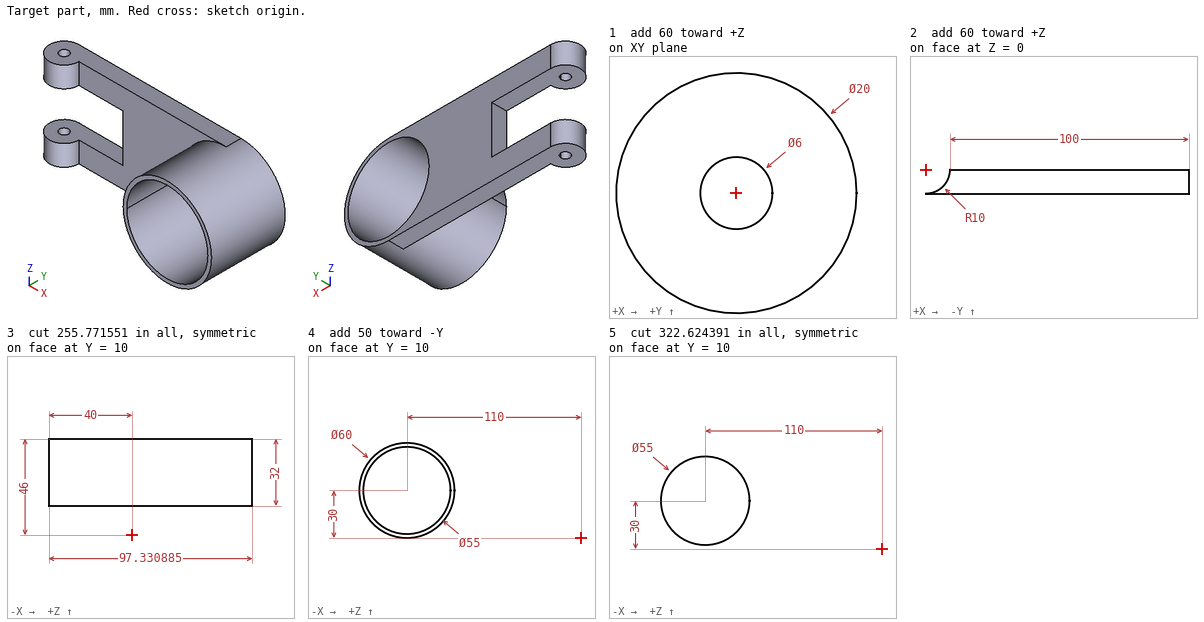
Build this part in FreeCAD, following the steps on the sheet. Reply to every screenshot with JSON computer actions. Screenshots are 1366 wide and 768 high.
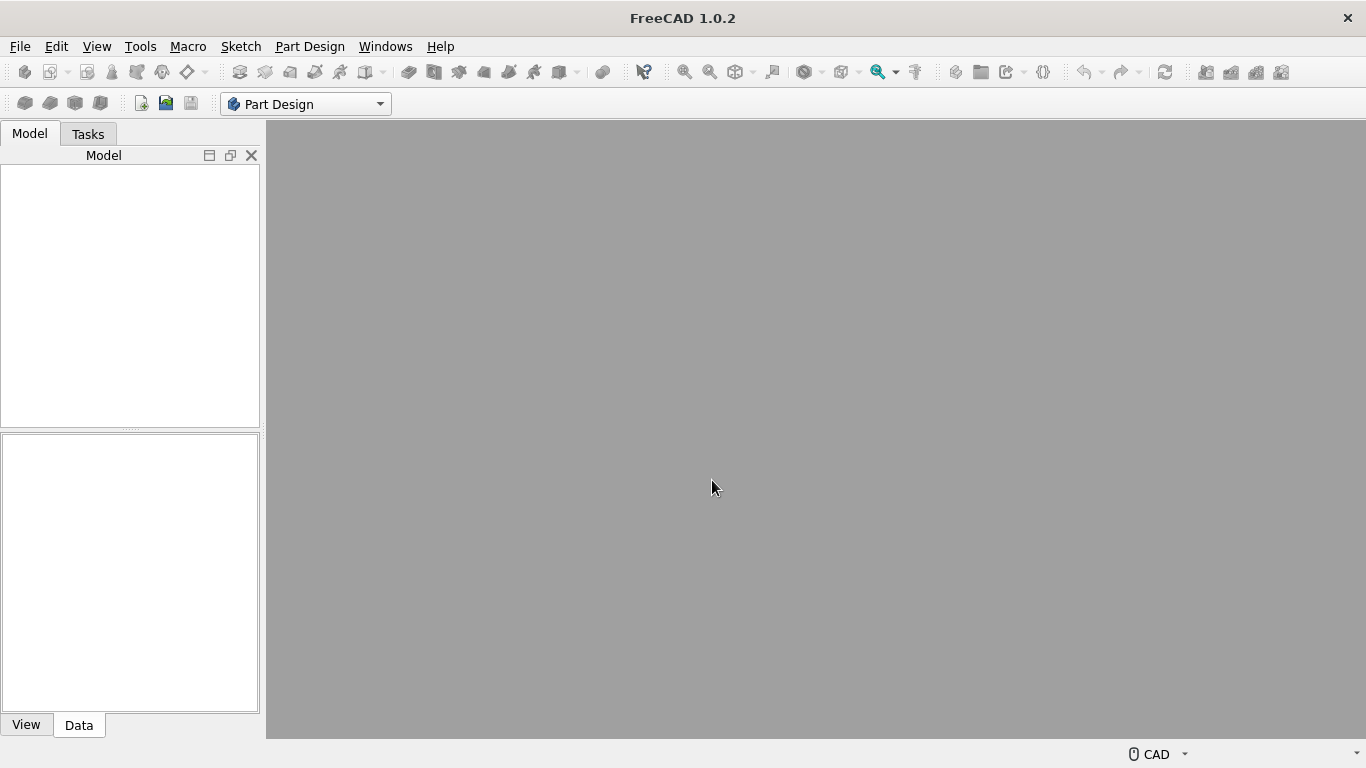
{"action": "left_click", "coordinate": [141, 104]}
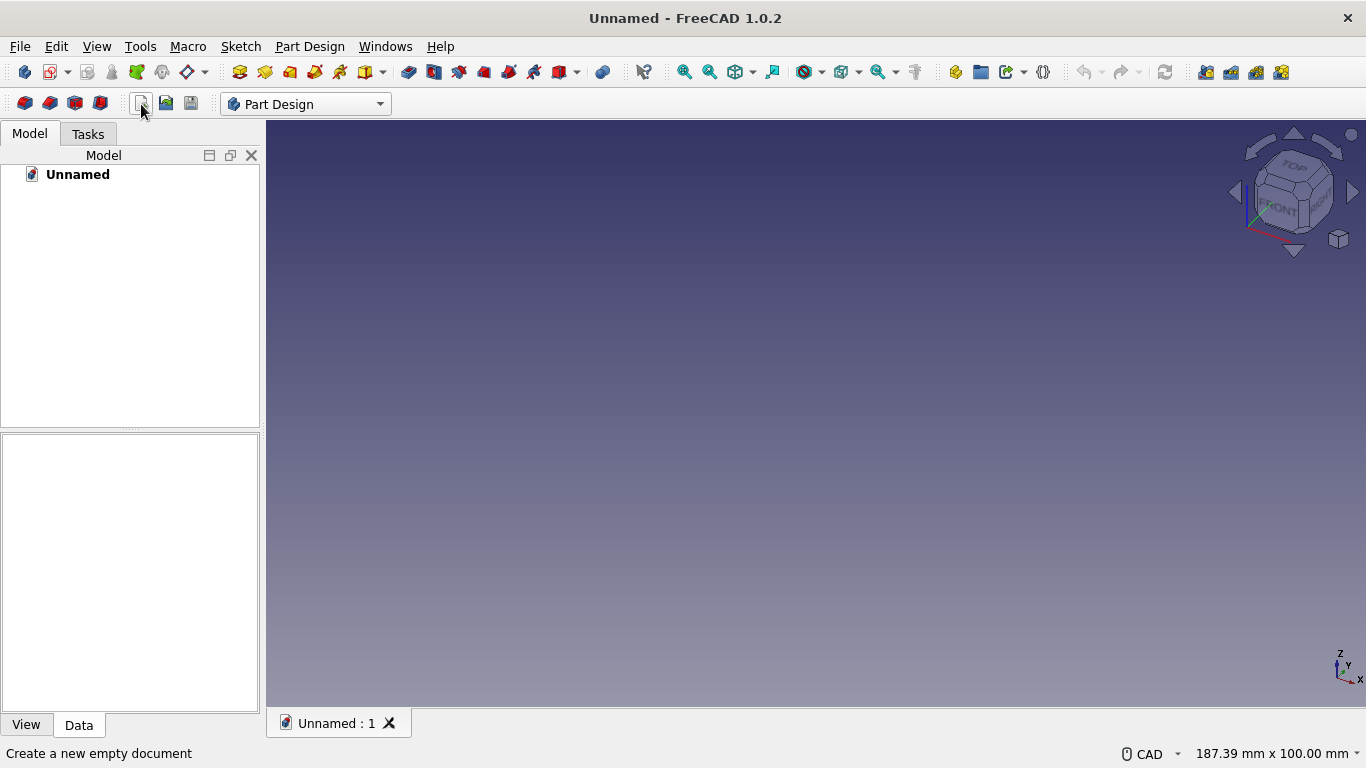
{"action": "left_click", "coordinate": [50, 72]}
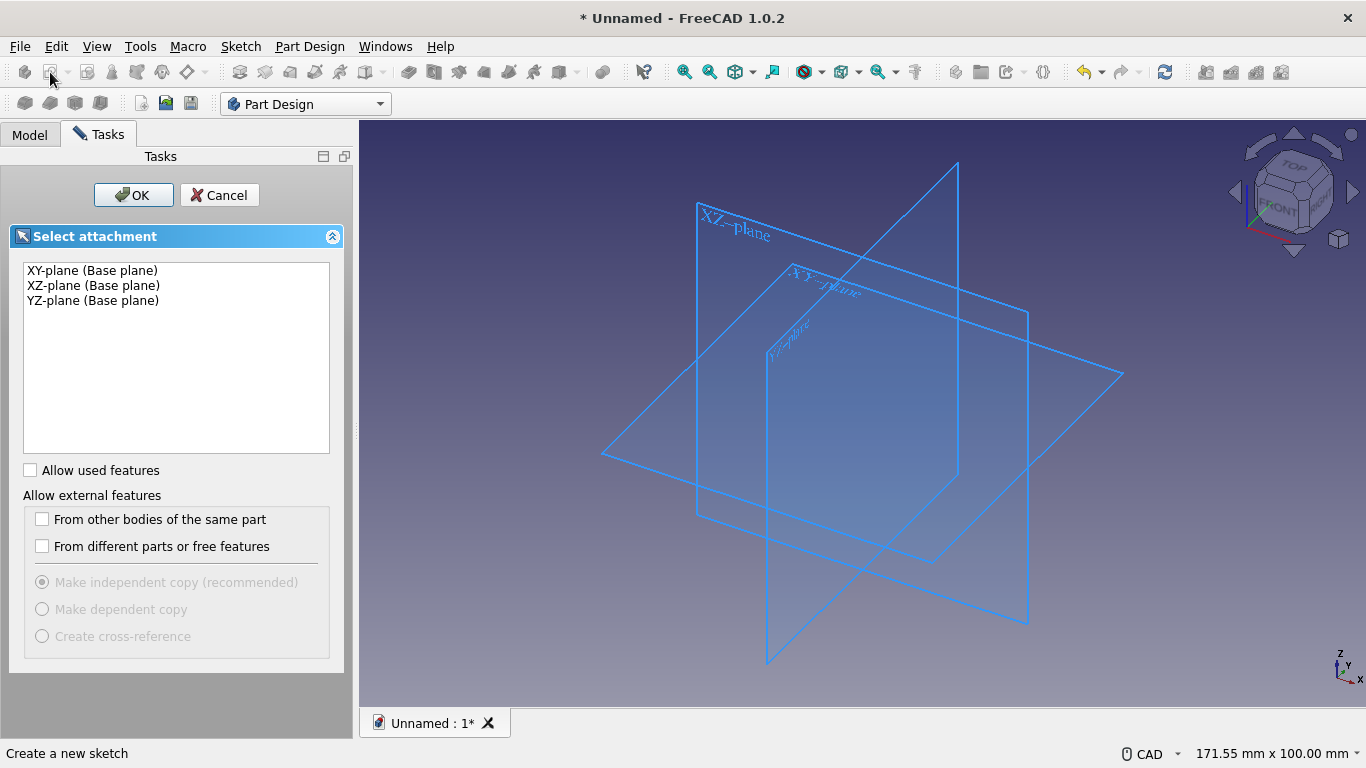
{"action": "left_click", "coordinate": [84, 270]}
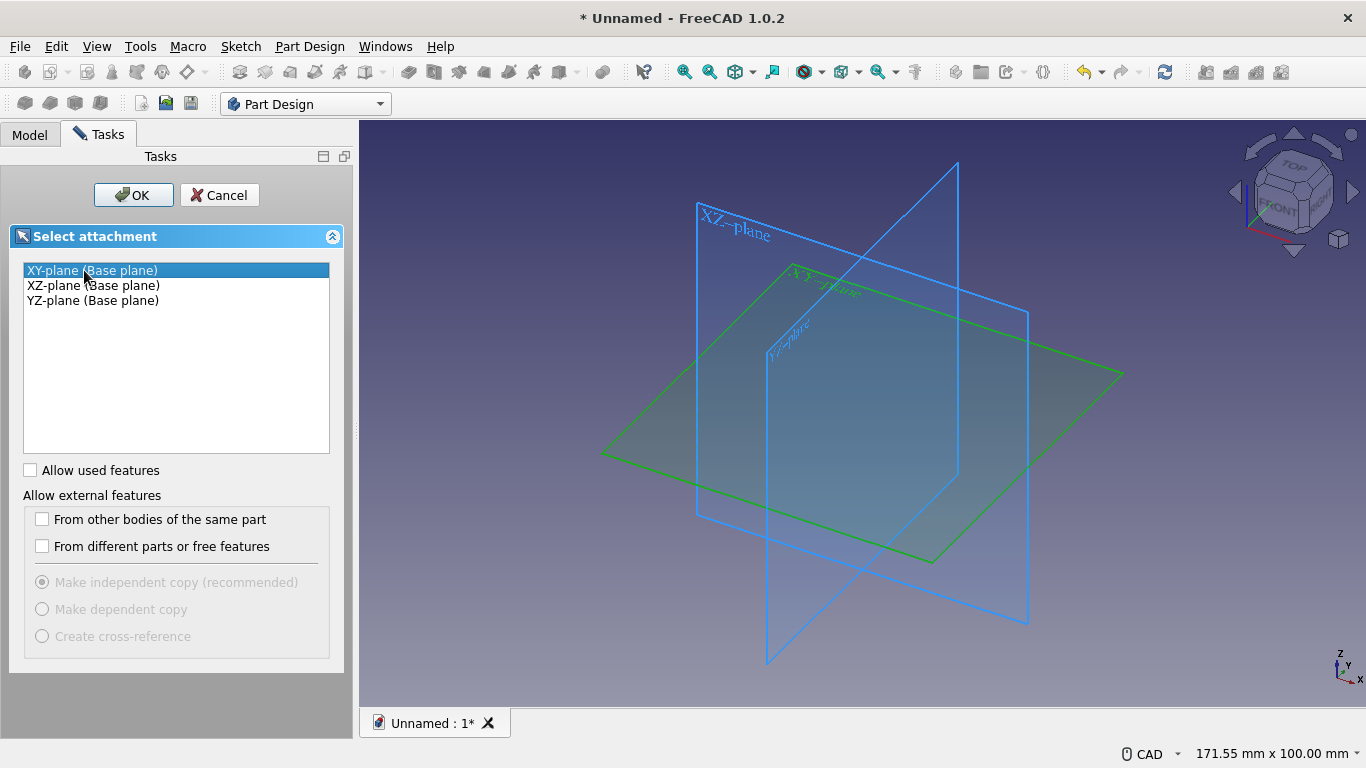
{"action": "left_click", "coordinate": [134, 195]}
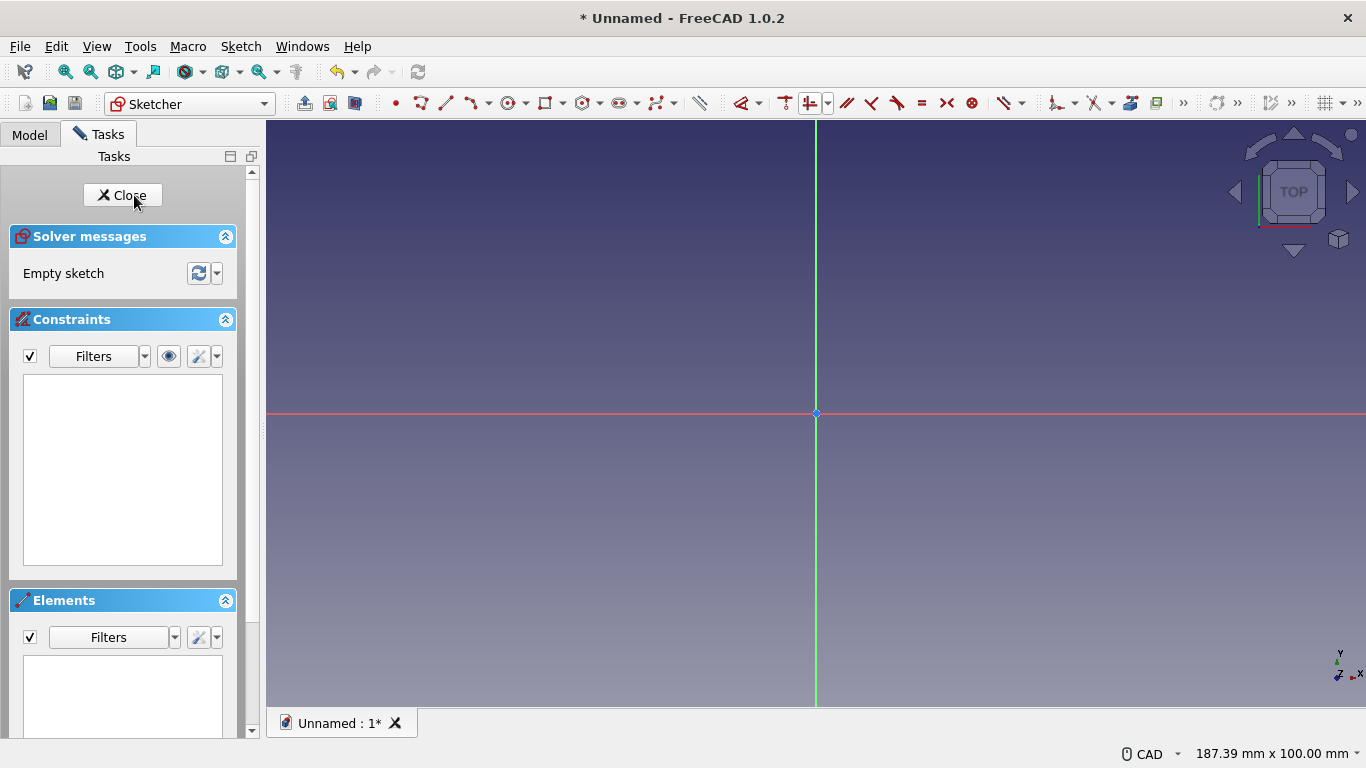
{"action": "scroll", "coordinate": [846, 414], "scroll_direction": "up", "scroll_amount": 6}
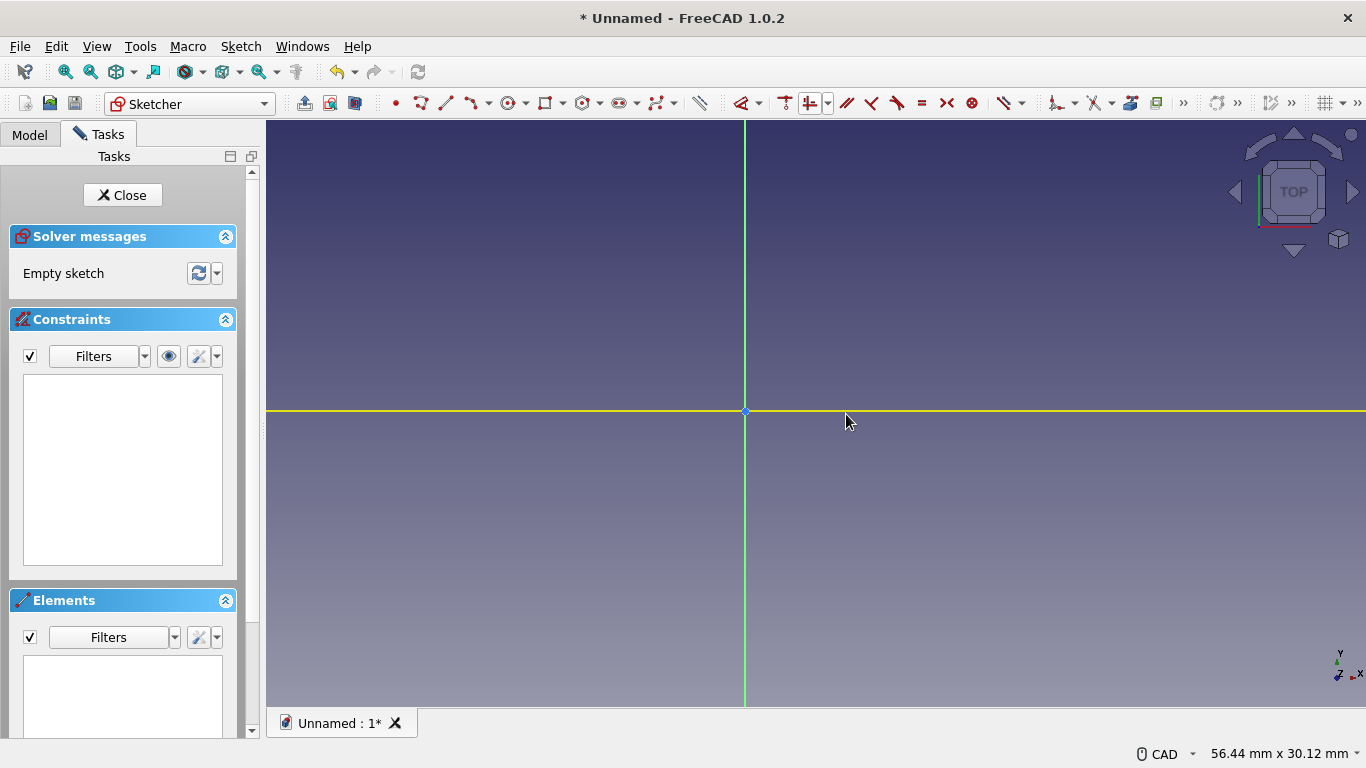
{"action": "left_click", "coordinate": [508, 104]}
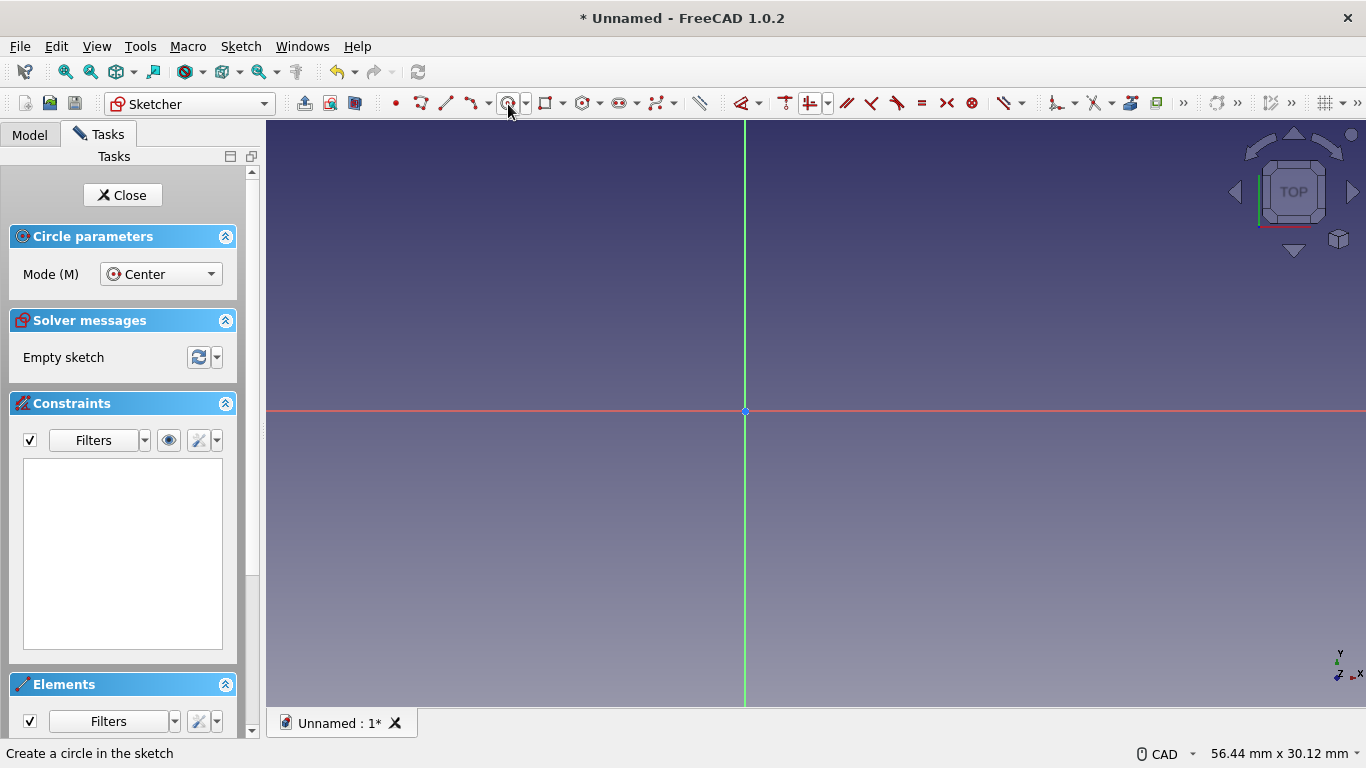
{"action": "left_click", "coordinate": [745, 411]}
{"action": "mouse_move", "coordinate": [883, 273]}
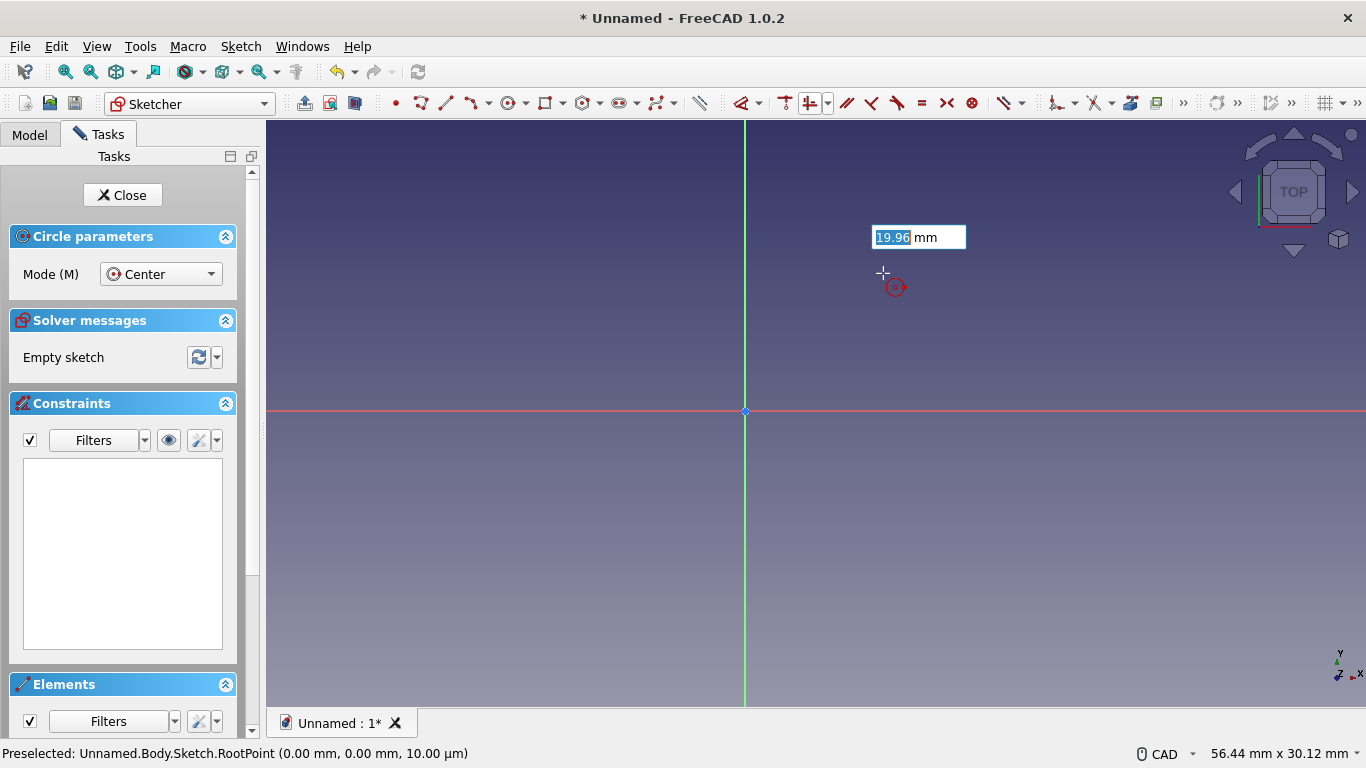
{"action": "type", "text": "20"}
{"action": "key", "text": "Return"}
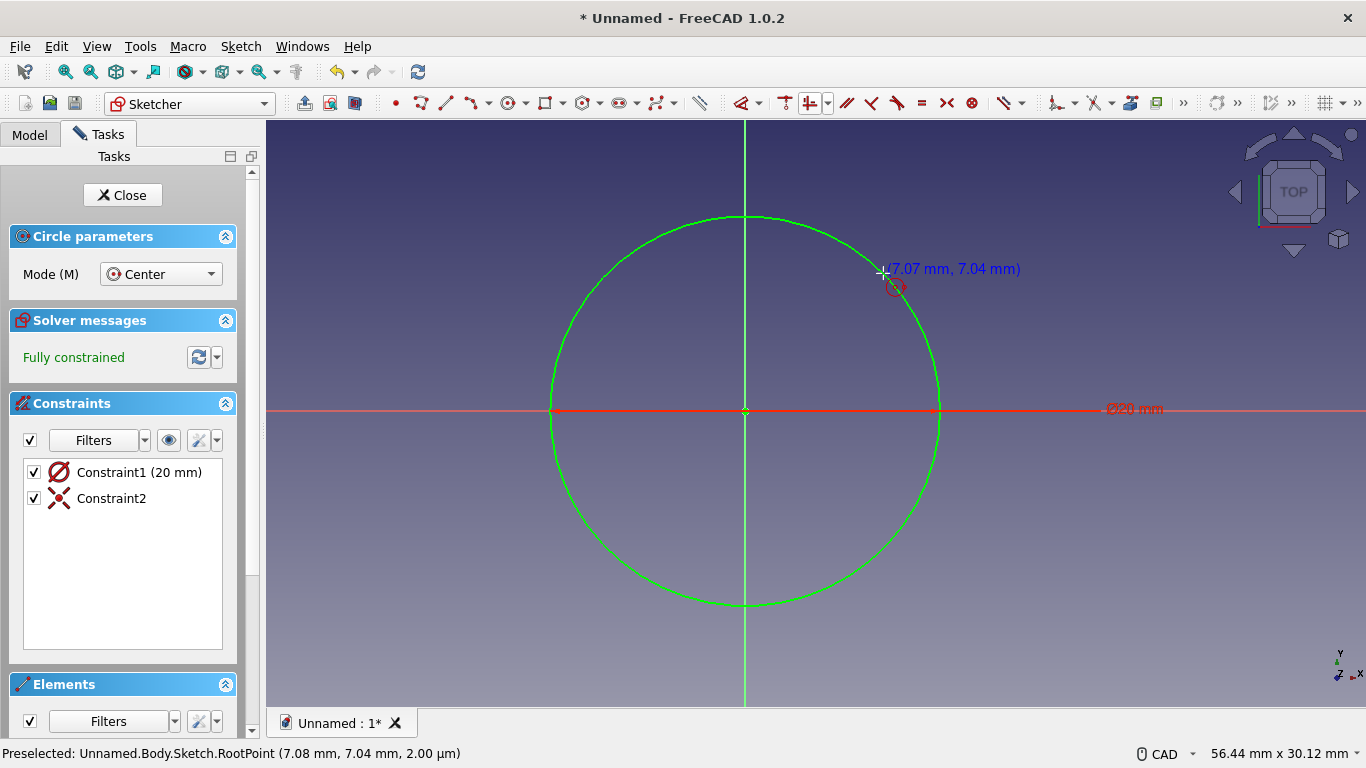
{"action": "left_click", "coordinate": [745, 411]}
{"action": "mouse_move", "coordinate": [787, 370]}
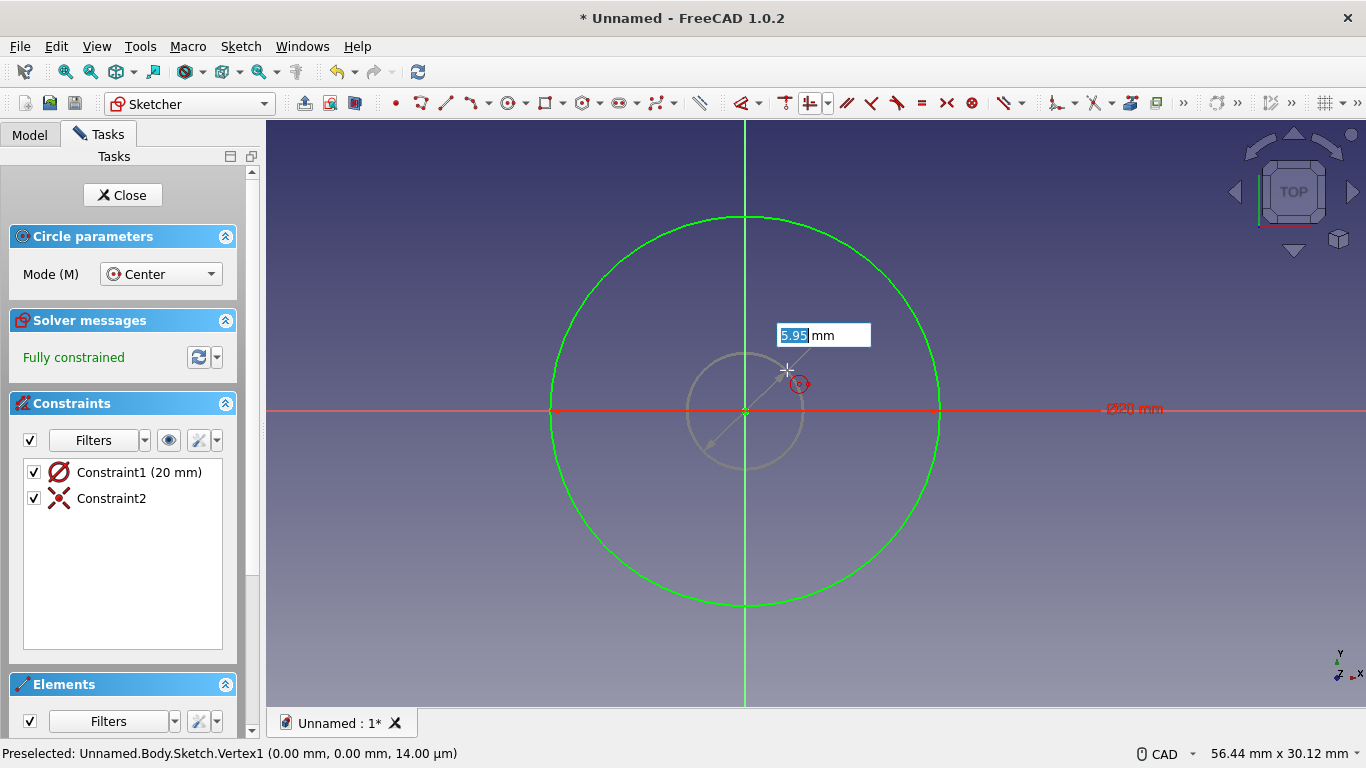
{"action": "type", "text": "6"}
{"action": "key", "text": "Return"}
{"action": "key", "text": "Escape"}